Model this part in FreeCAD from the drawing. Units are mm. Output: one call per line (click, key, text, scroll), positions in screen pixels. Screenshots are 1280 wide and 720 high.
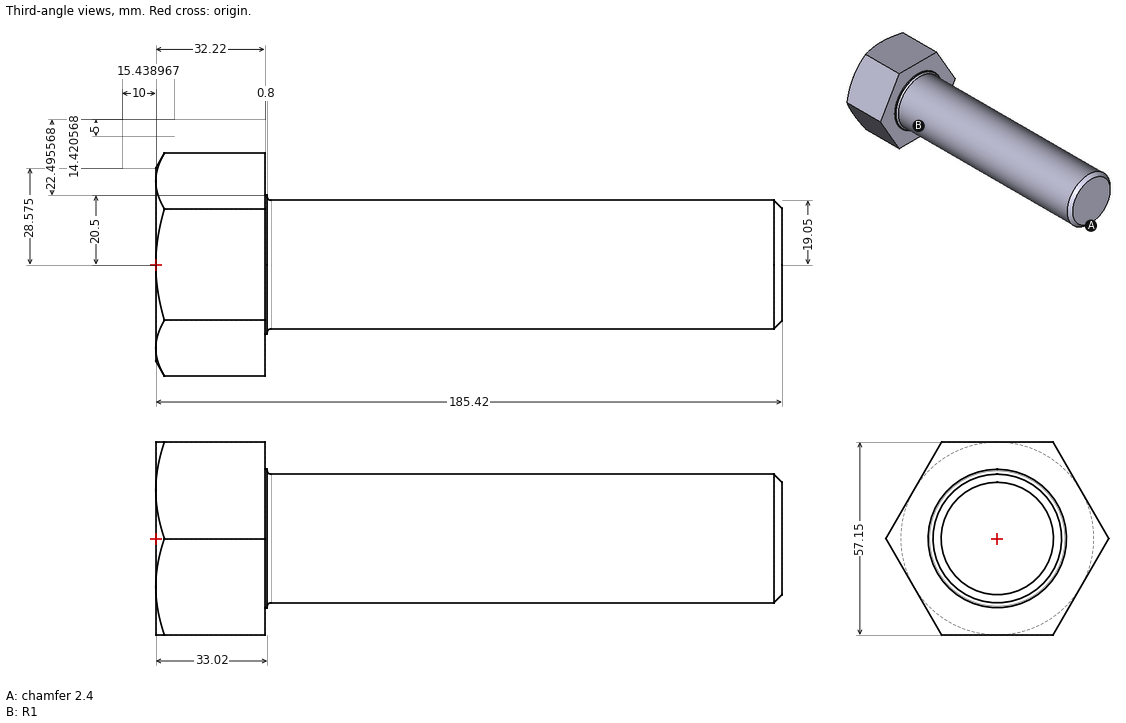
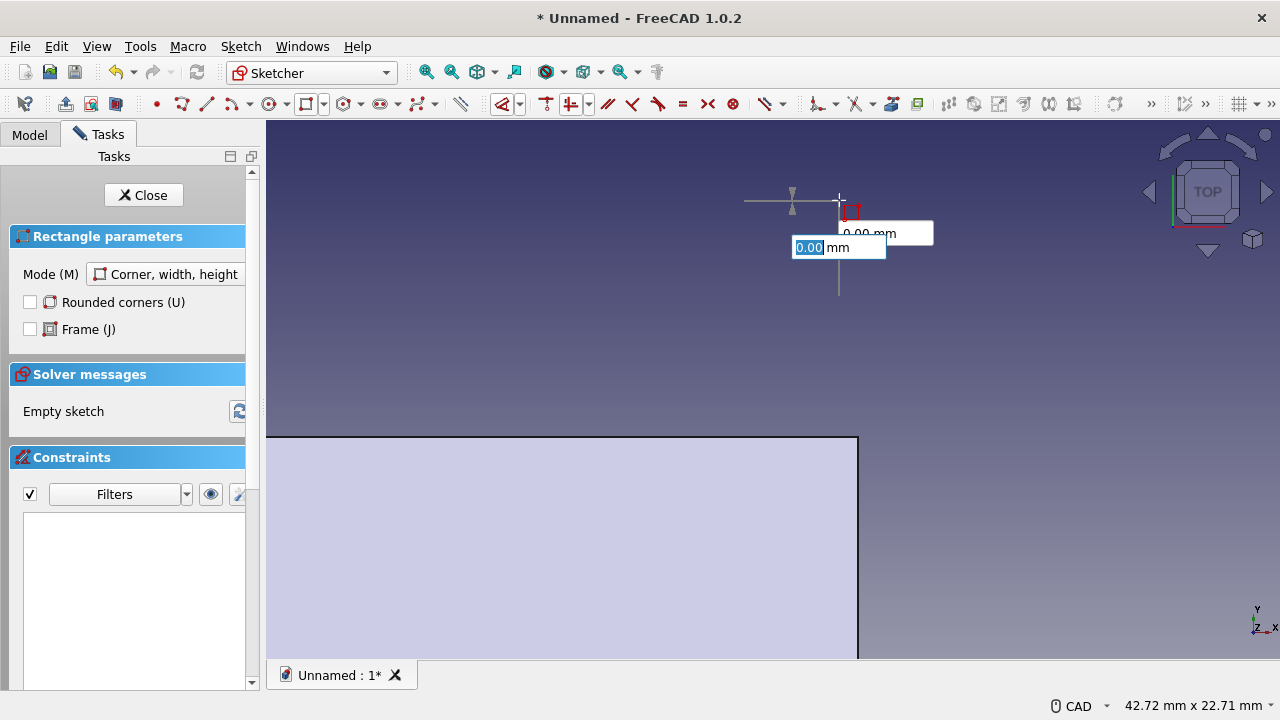
scroll(843, 203, down, 5)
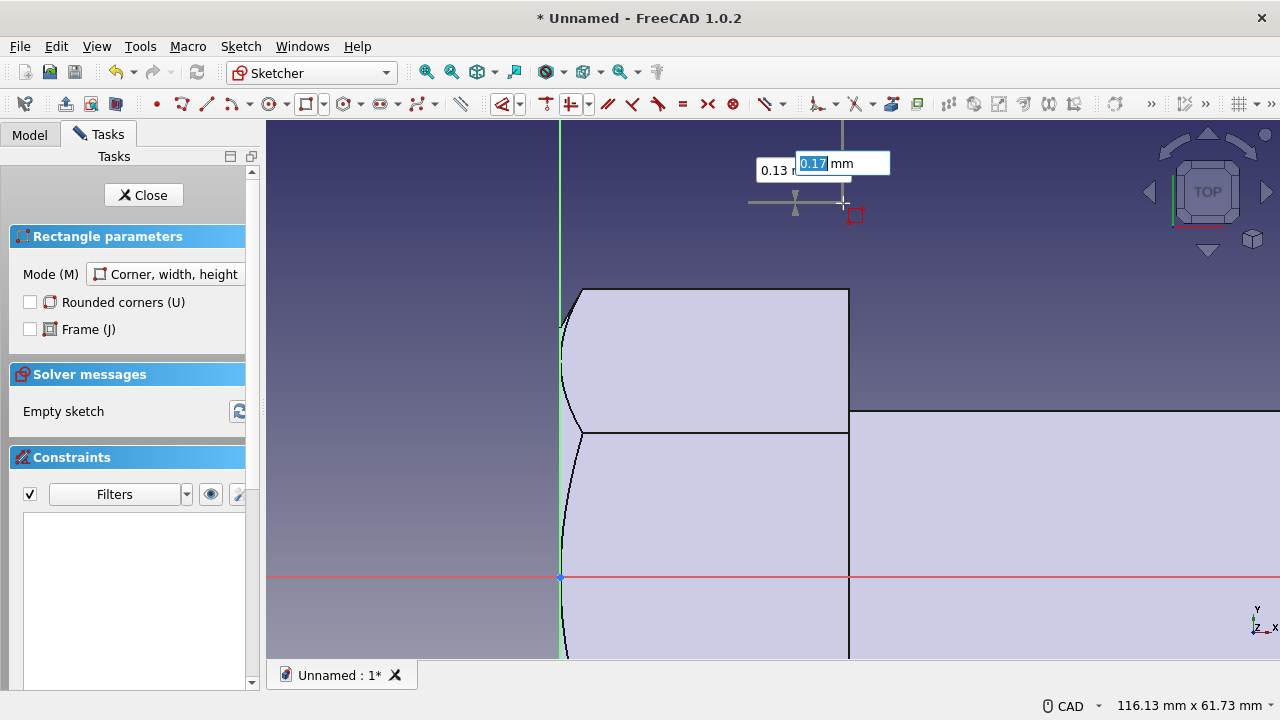
click(849, 398)
key(Escape)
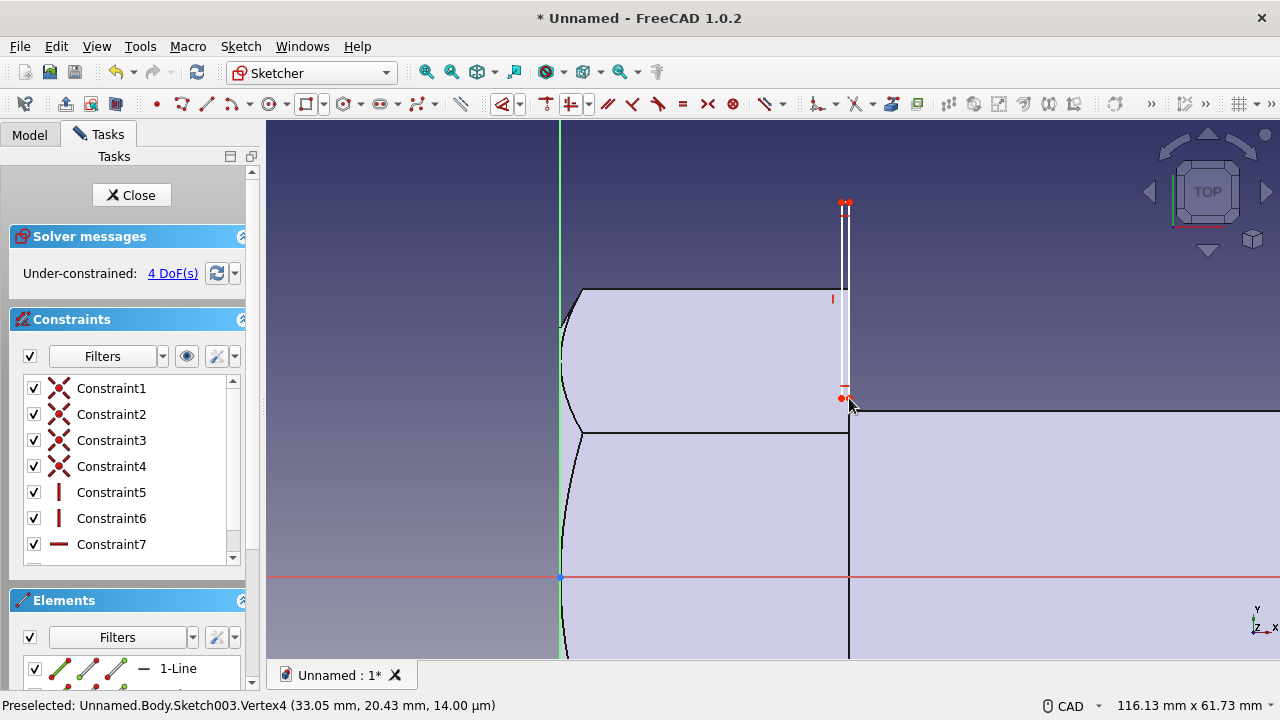
scroll(845, 399, up, 9)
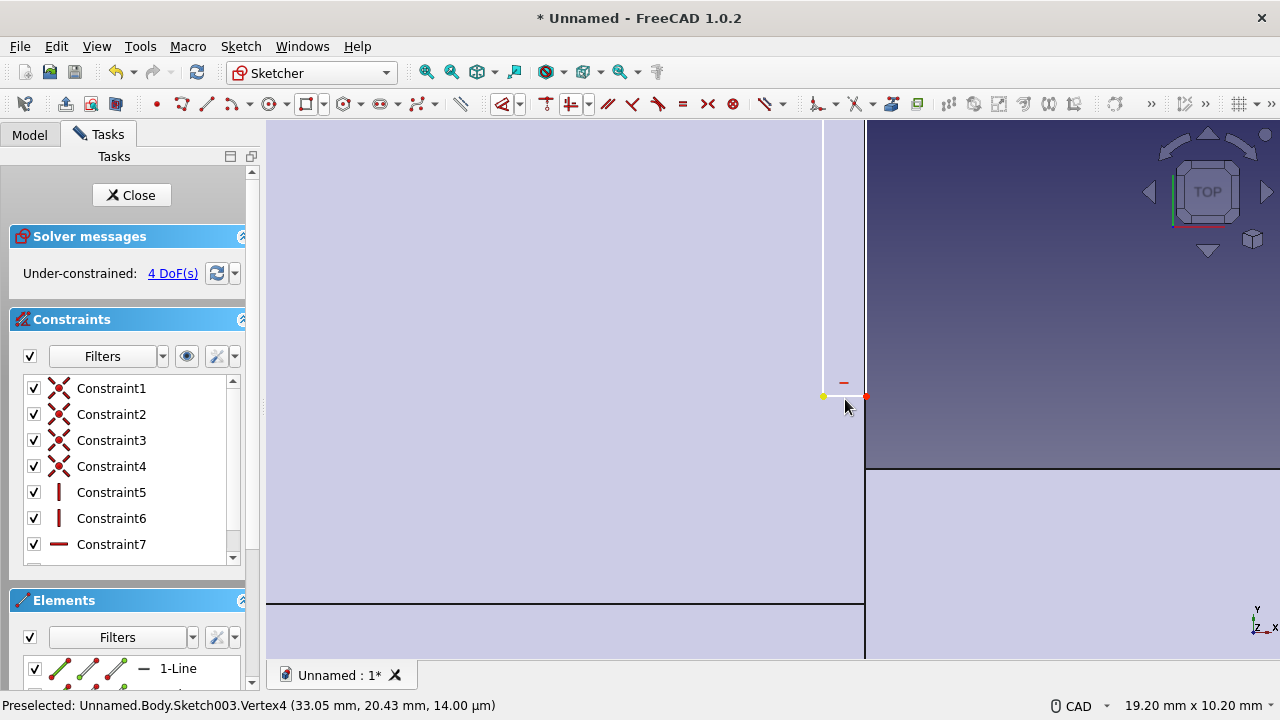
click(845, 396)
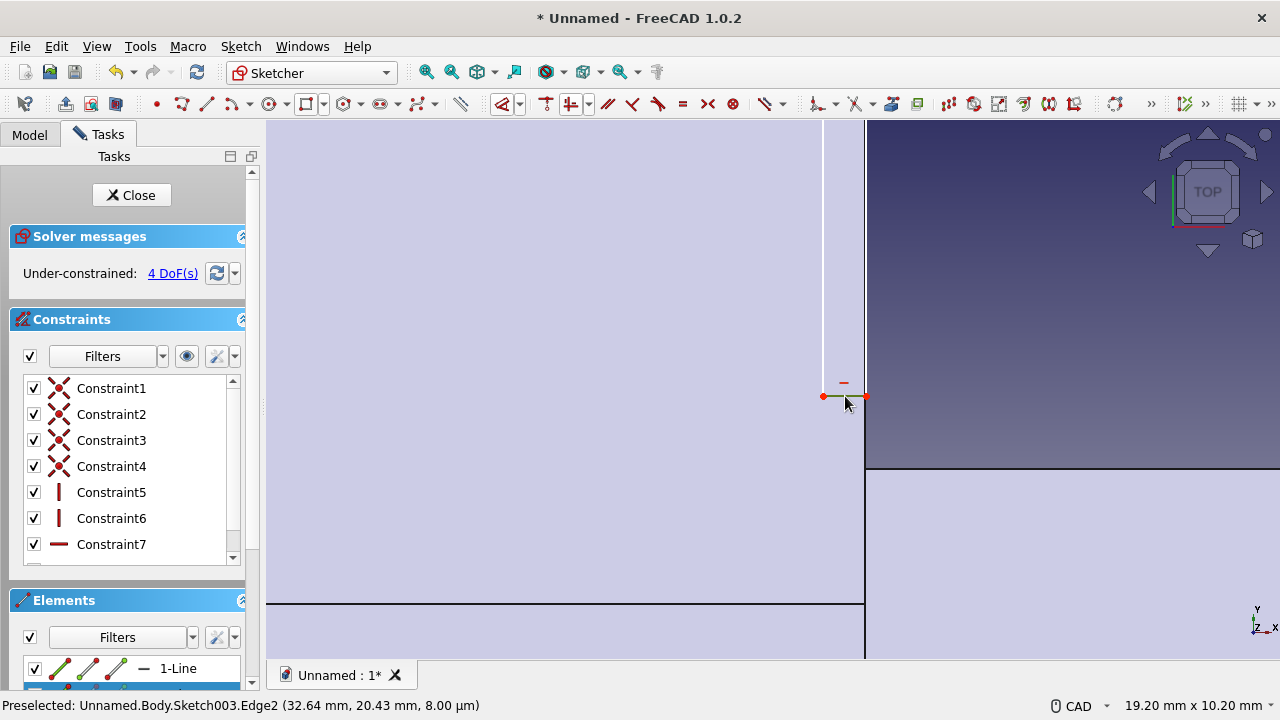
click(520, 104)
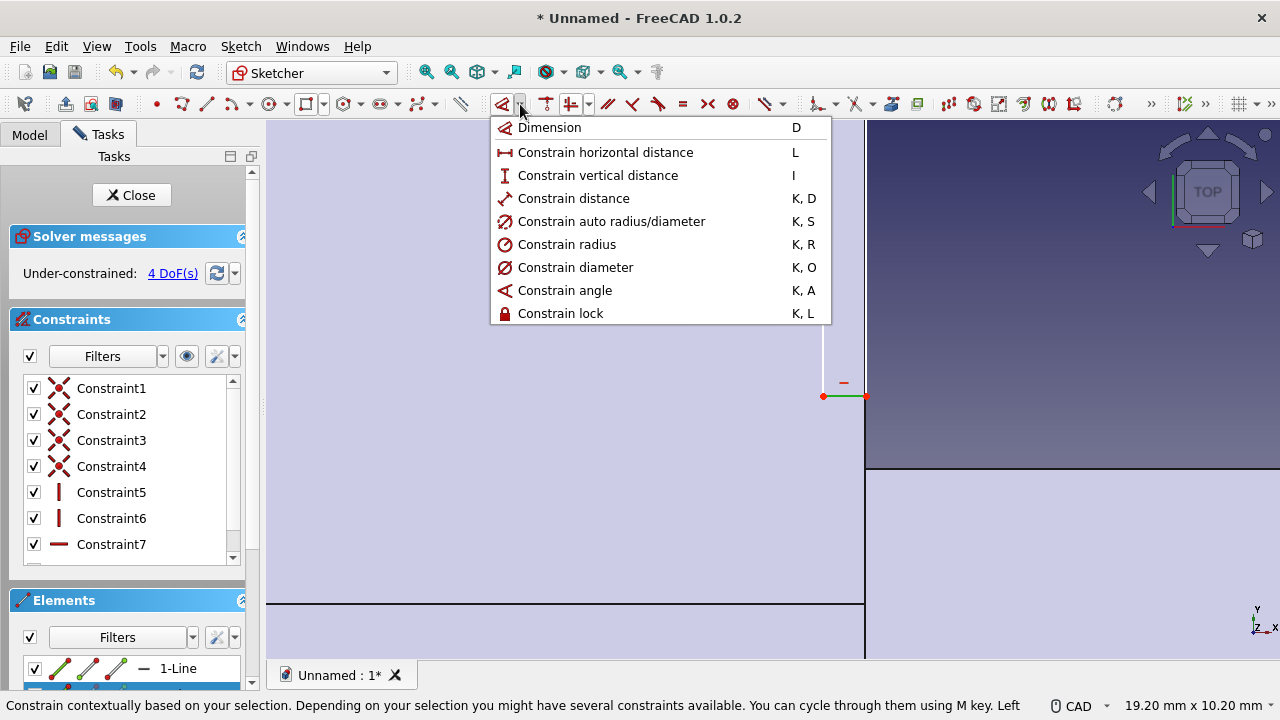
click(661, 152)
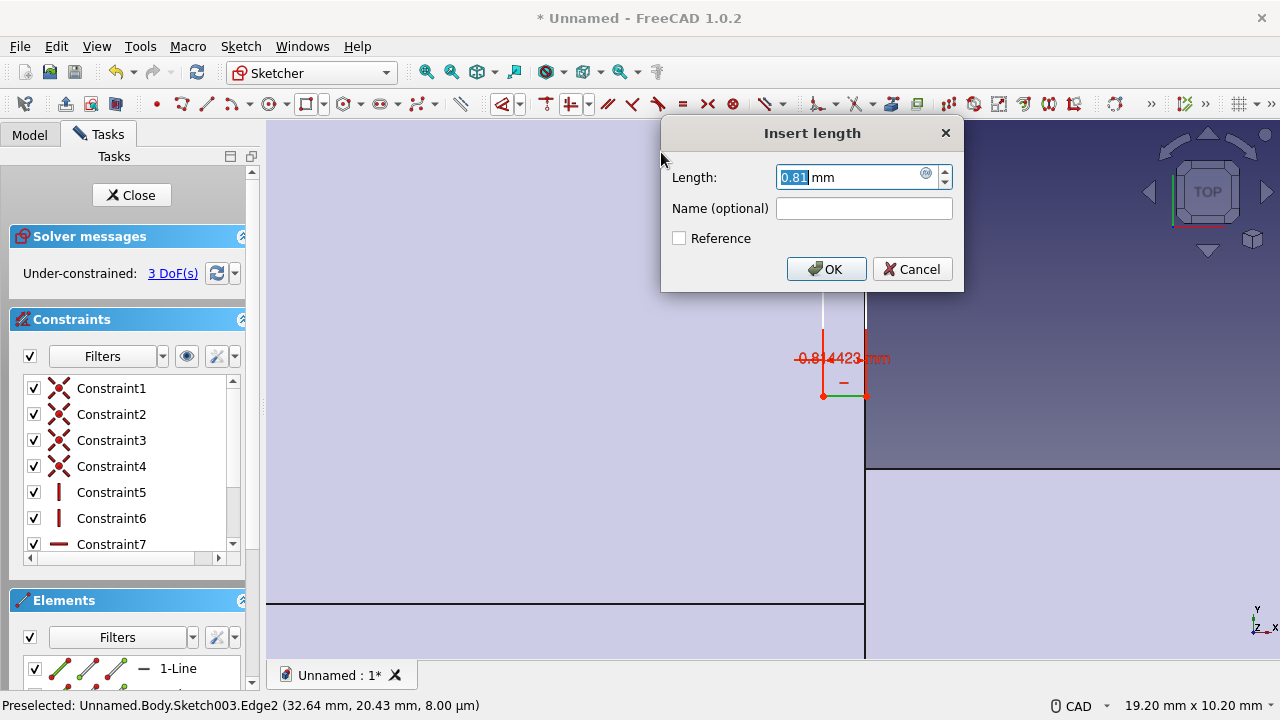
text(0.8)
key(Return)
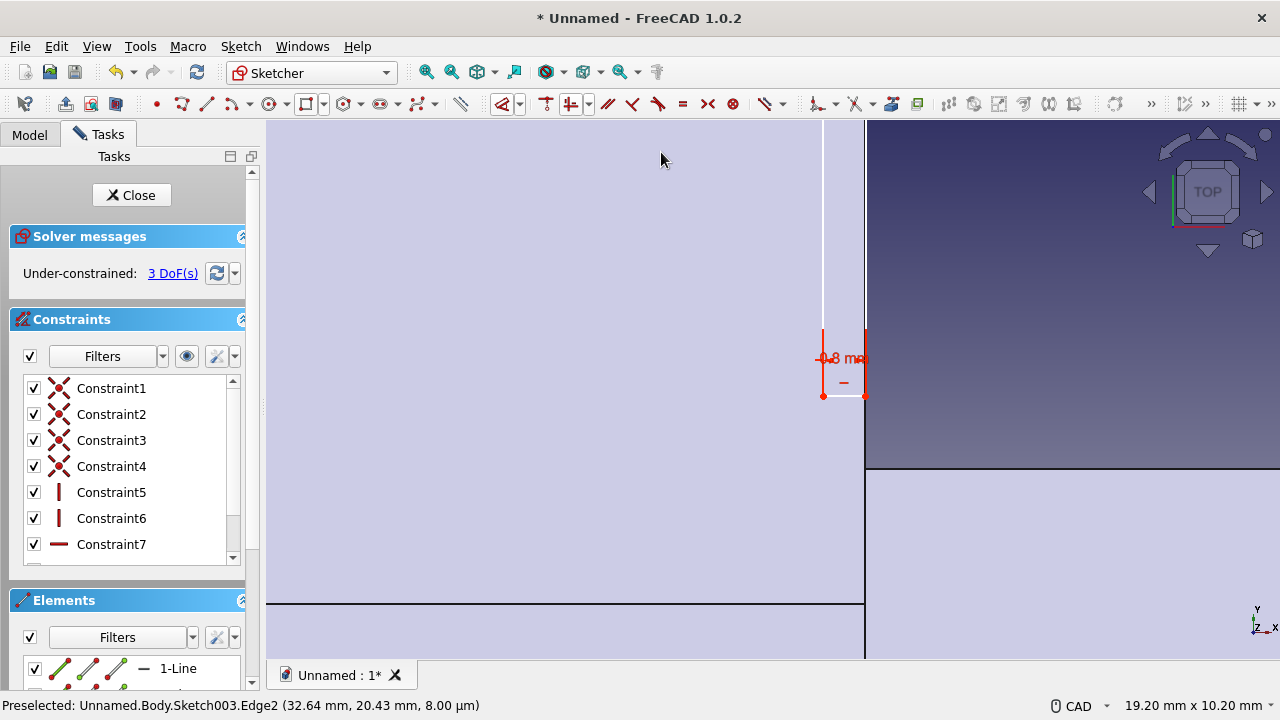
scroll(845, 399, down, 9)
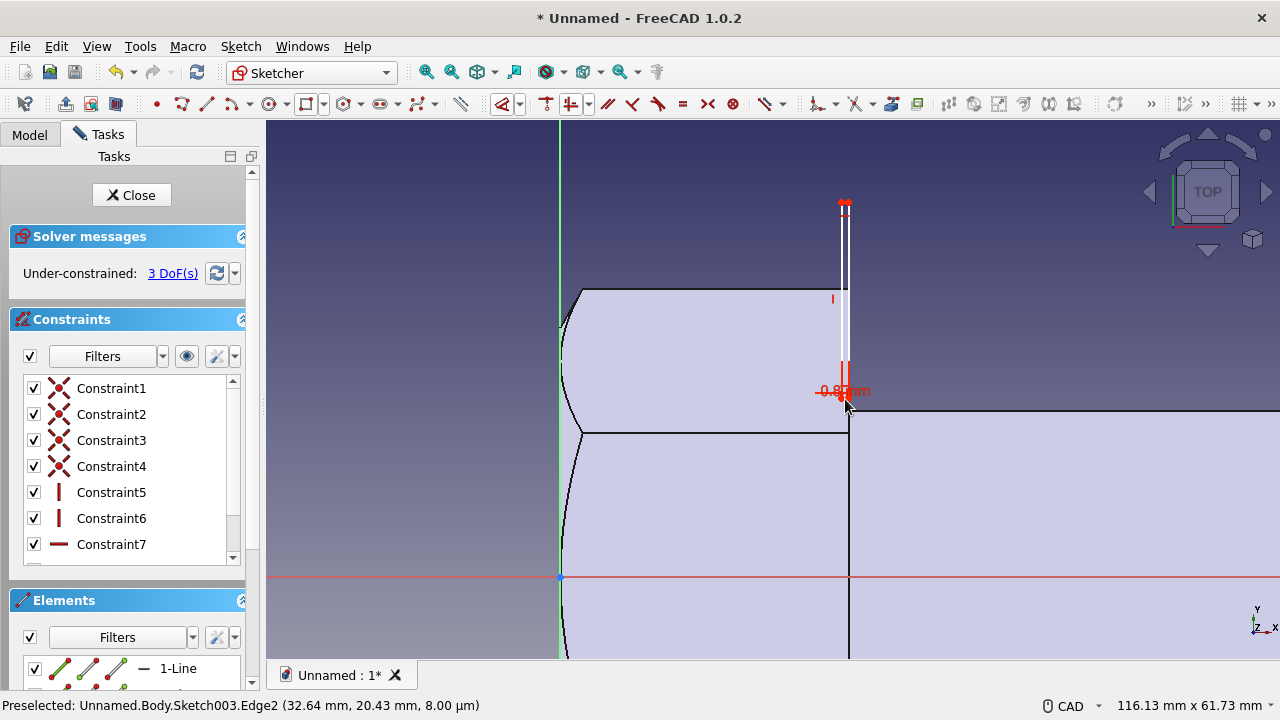
scroll(842, 399, up, 3)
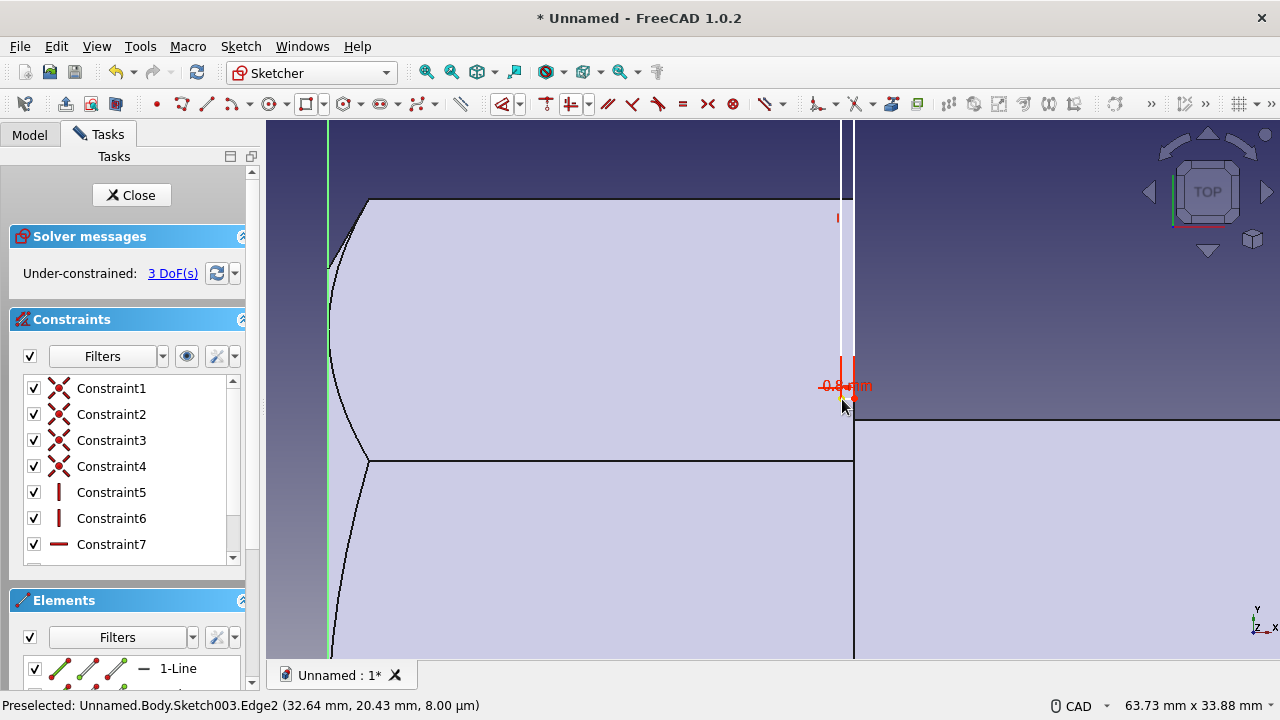
click(841, 399)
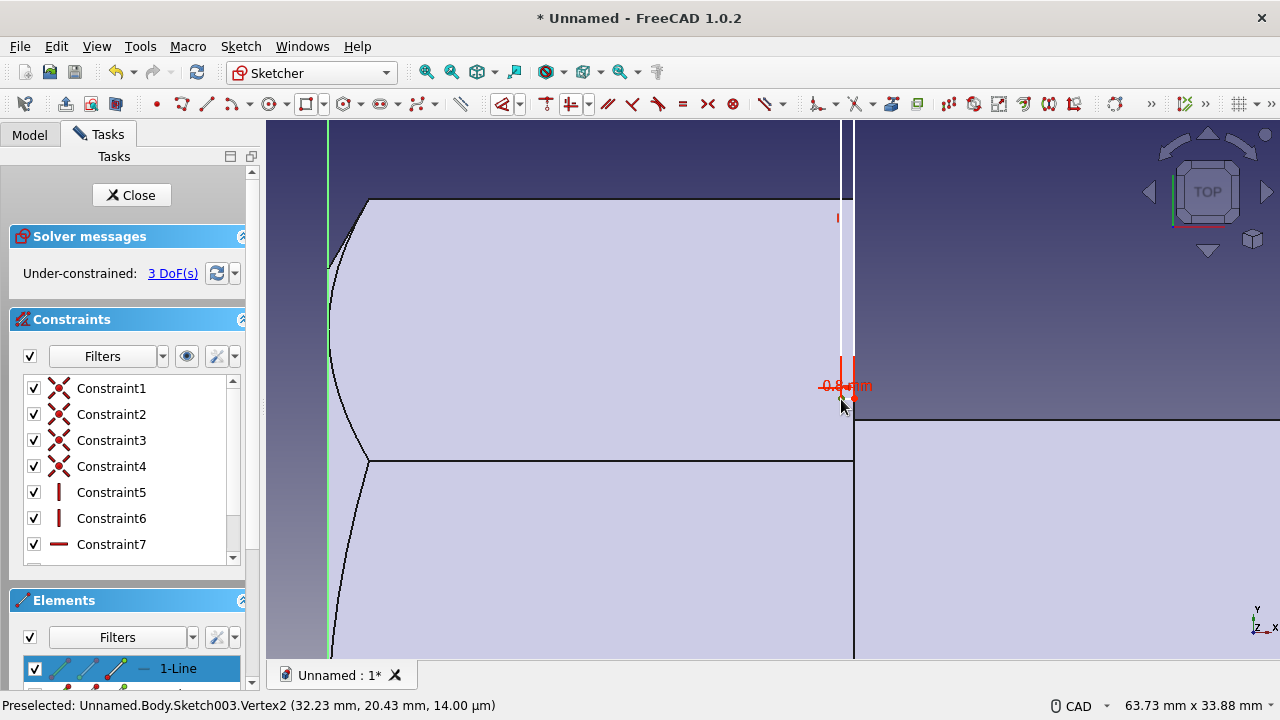
click(520, 104)